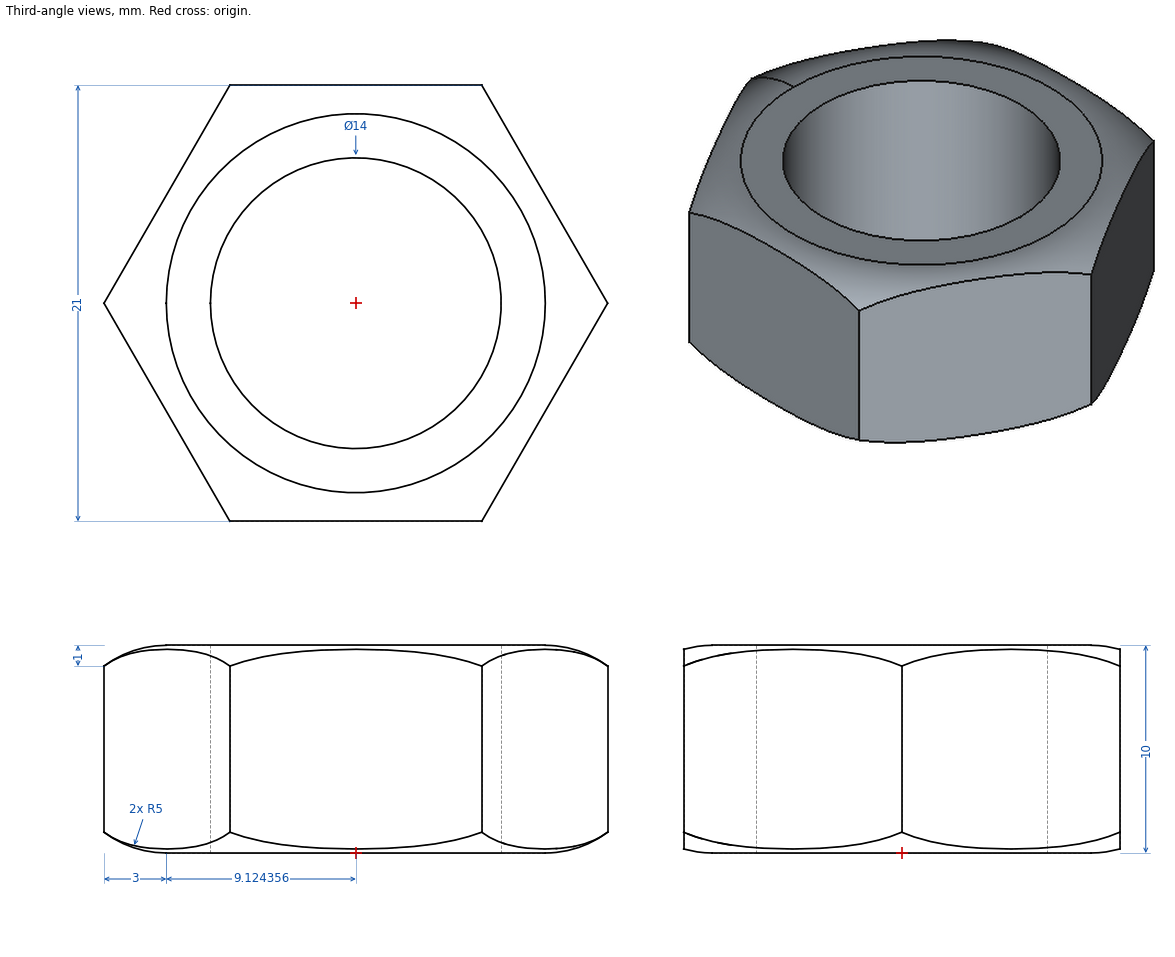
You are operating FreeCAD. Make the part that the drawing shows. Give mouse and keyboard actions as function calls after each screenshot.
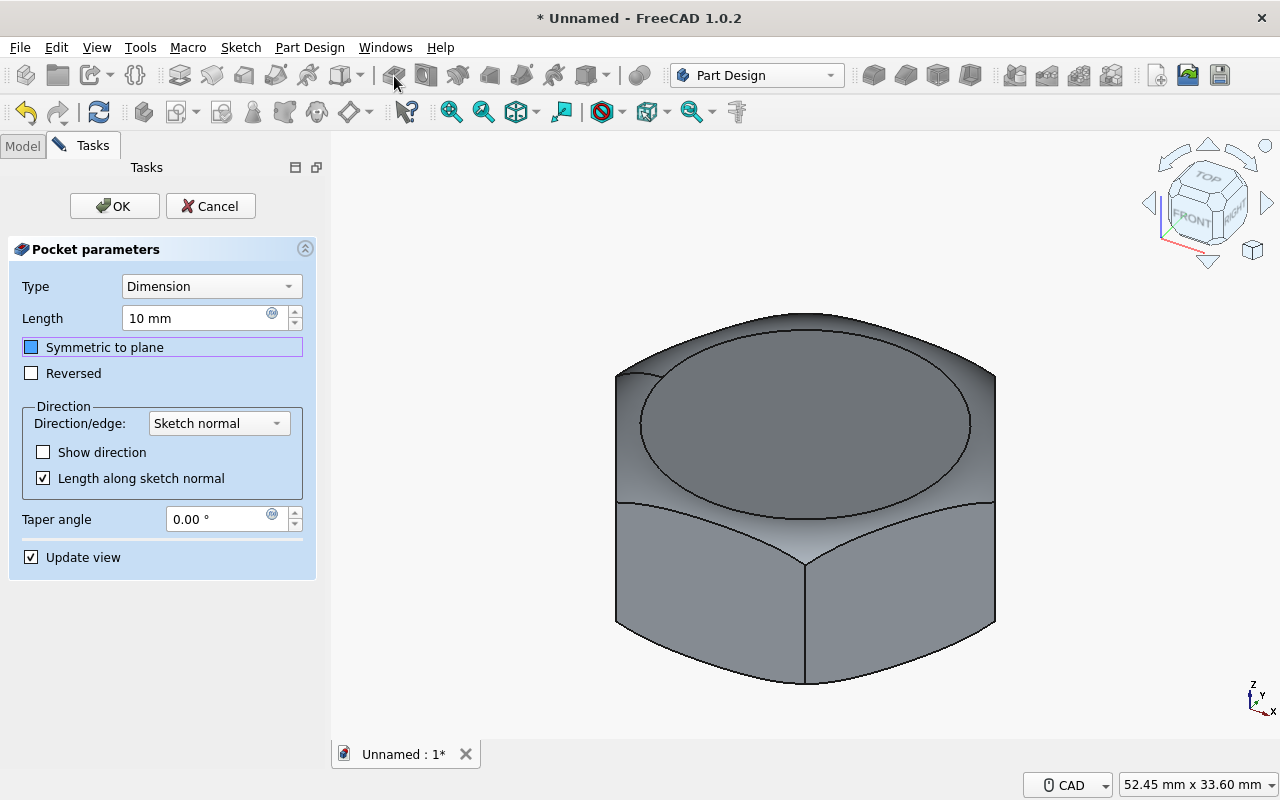
click(30, 373)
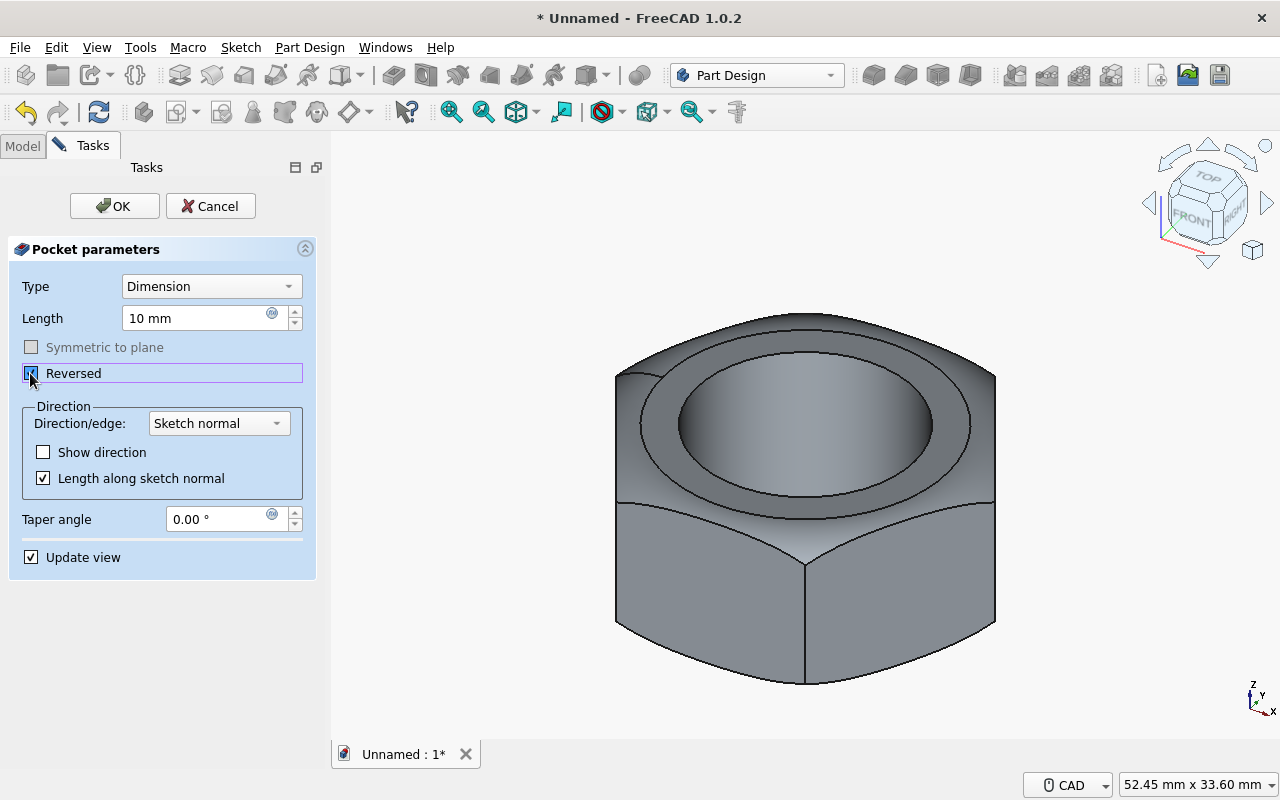
click(115, 206)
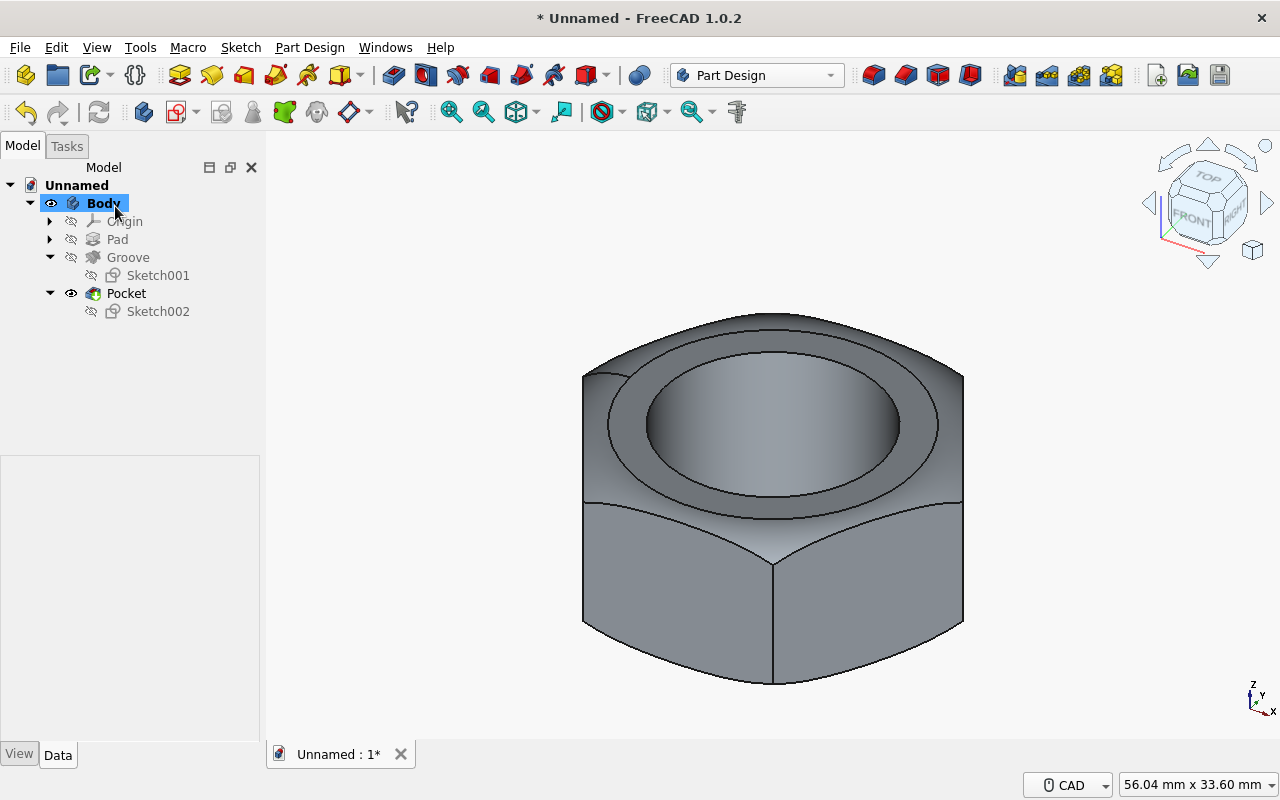
key(0)